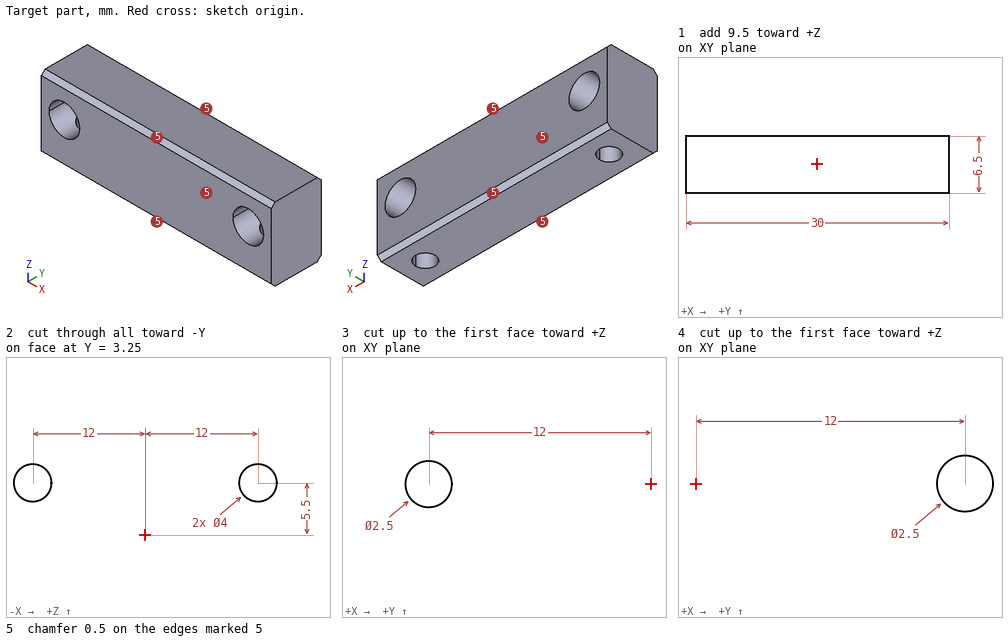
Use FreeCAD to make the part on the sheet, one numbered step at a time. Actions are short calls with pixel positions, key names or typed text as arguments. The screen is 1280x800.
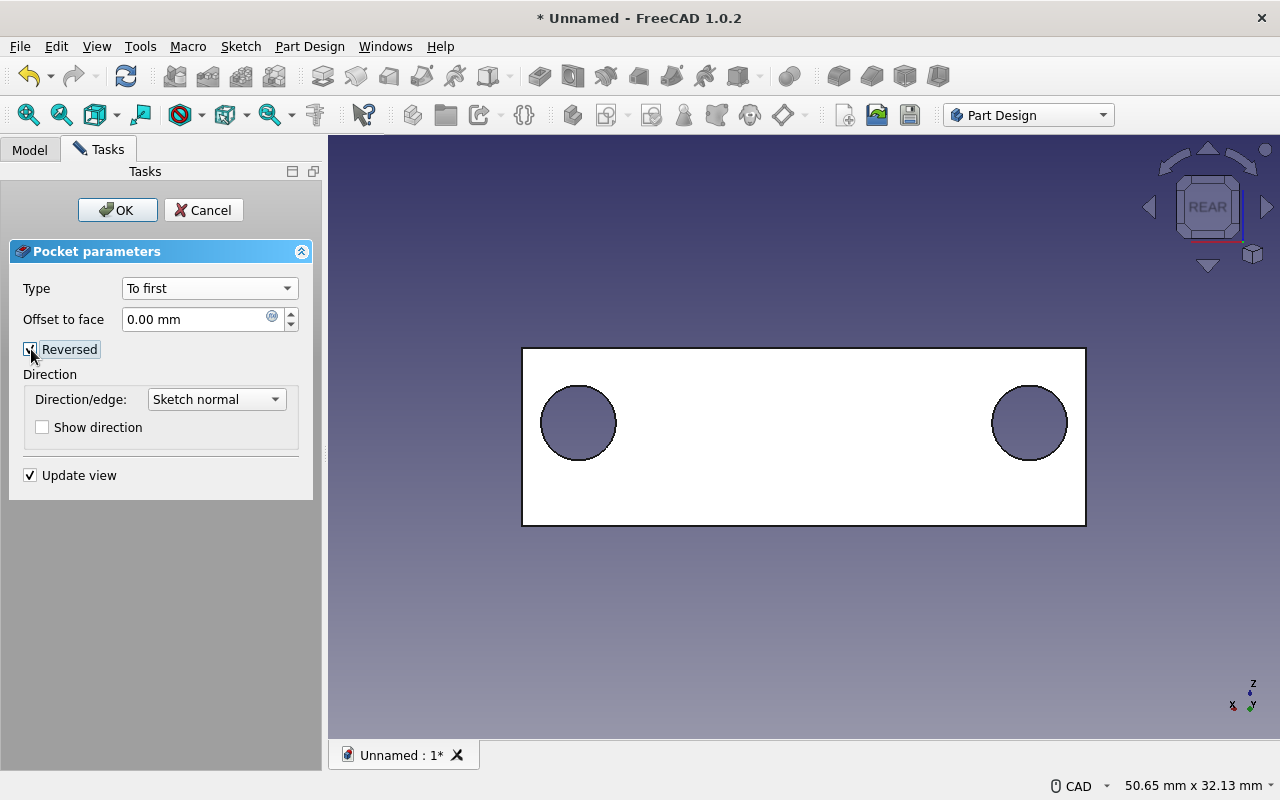
click(118, 210)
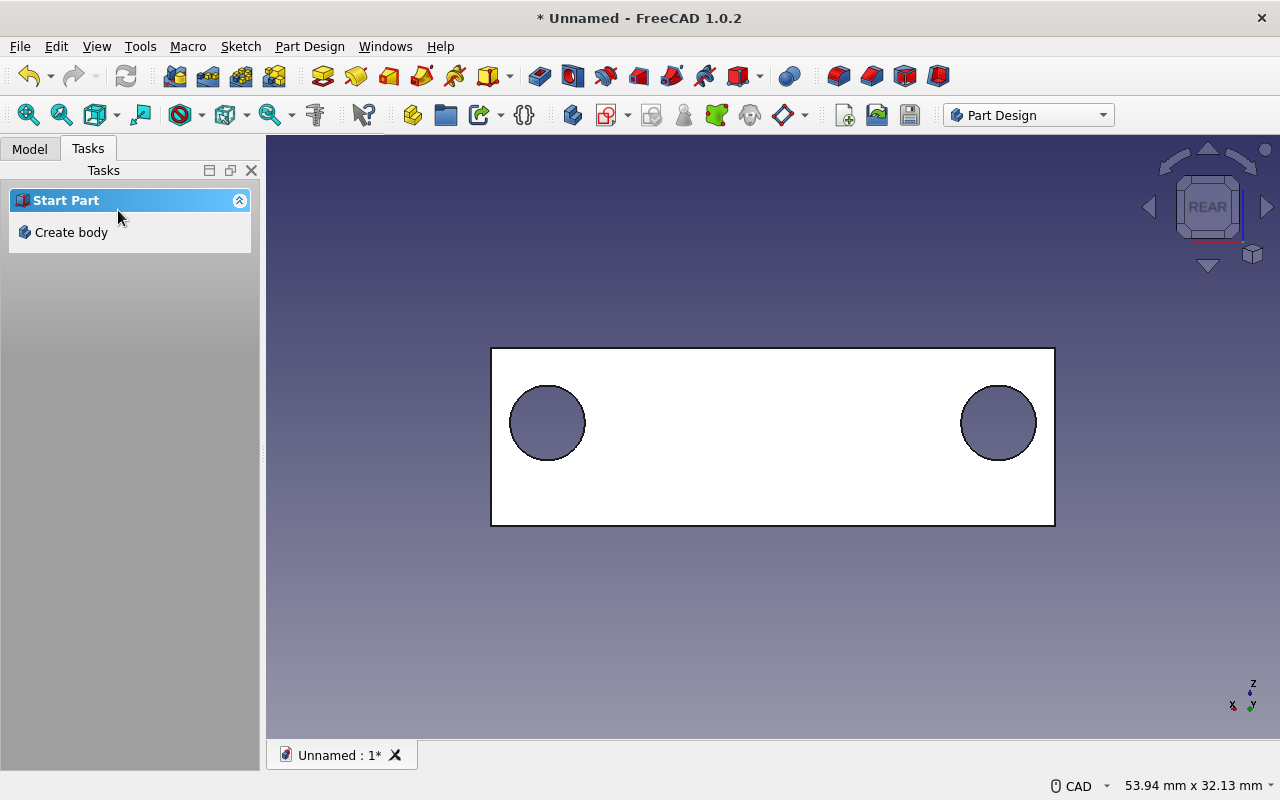
click(606, 116)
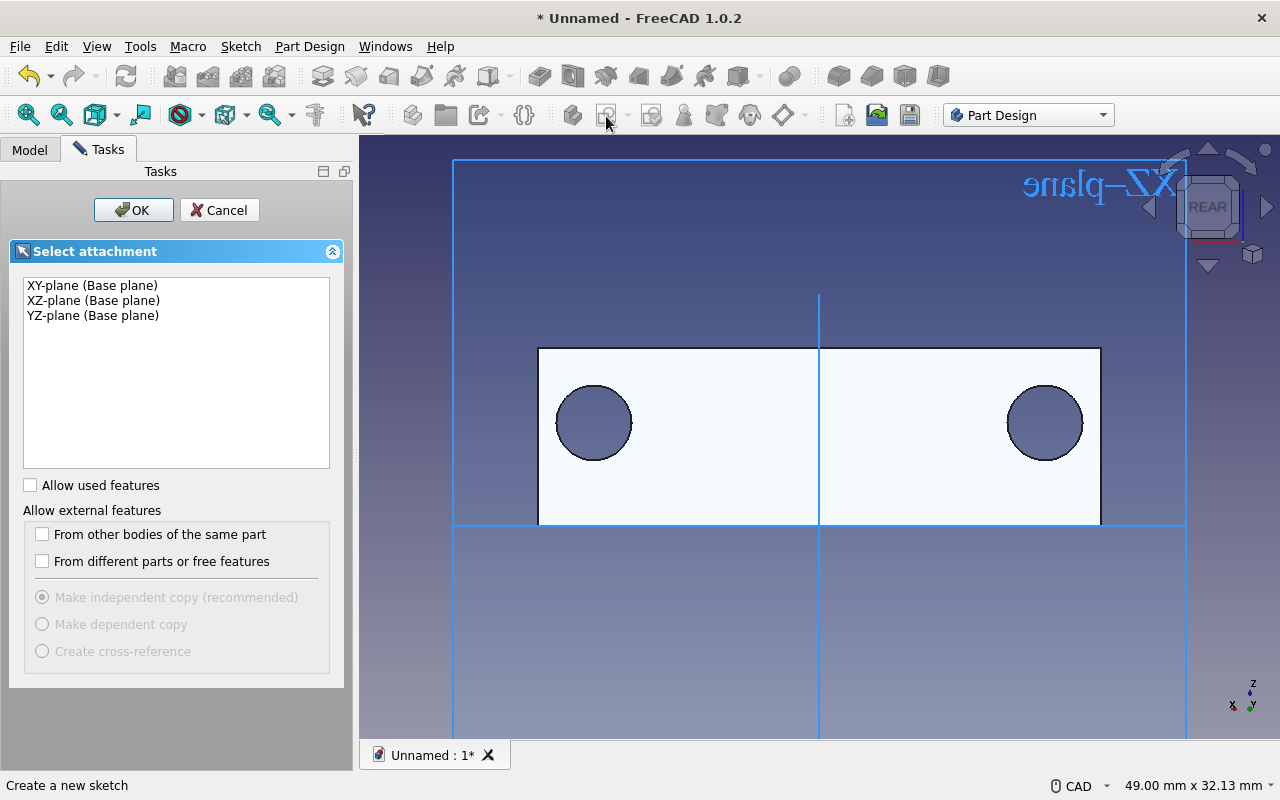
click(84, 286)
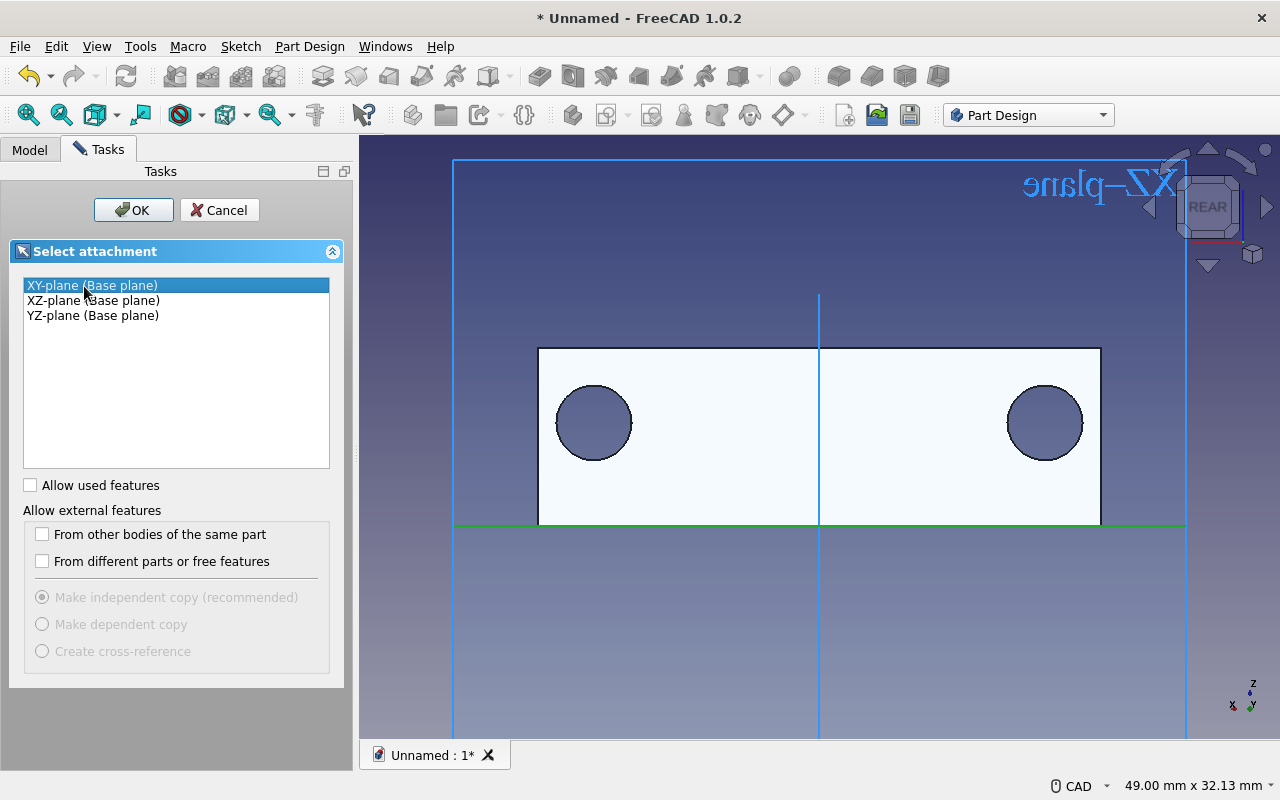
click(134, 210)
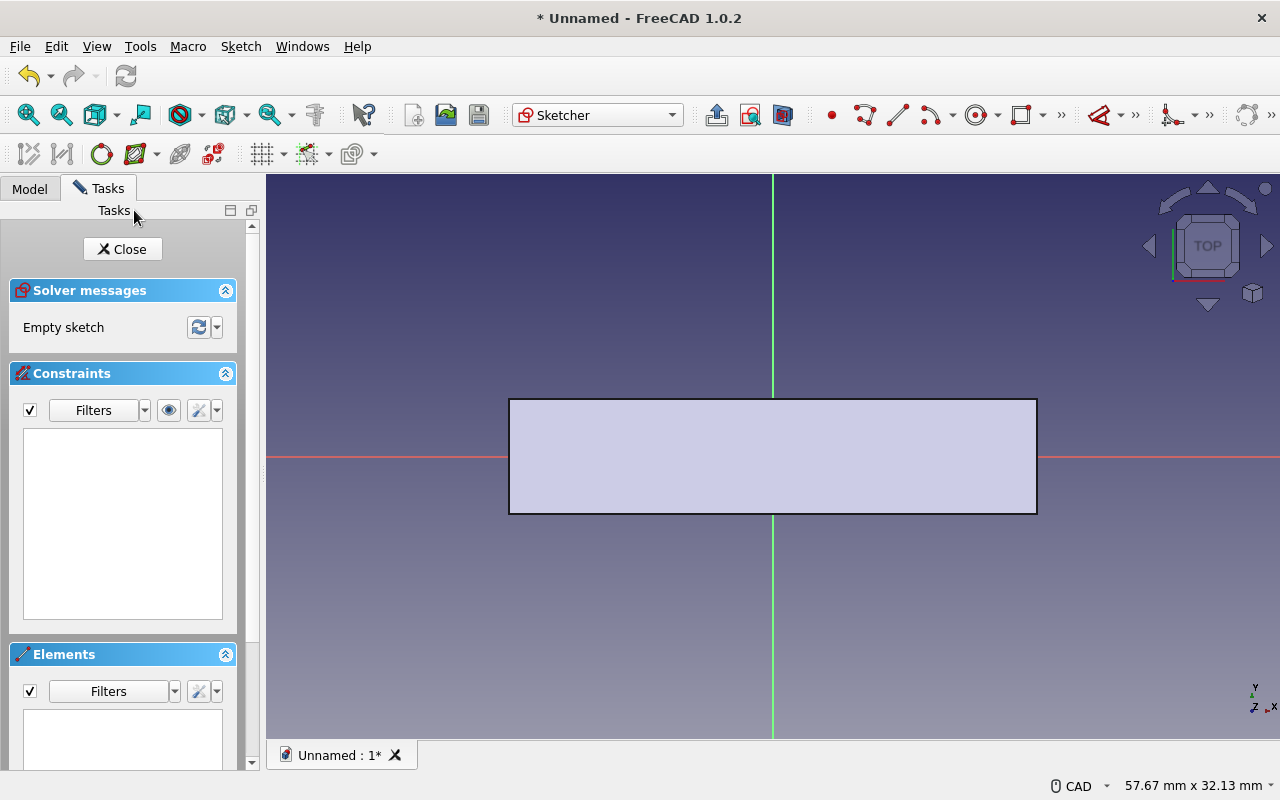
key(q)
key(s)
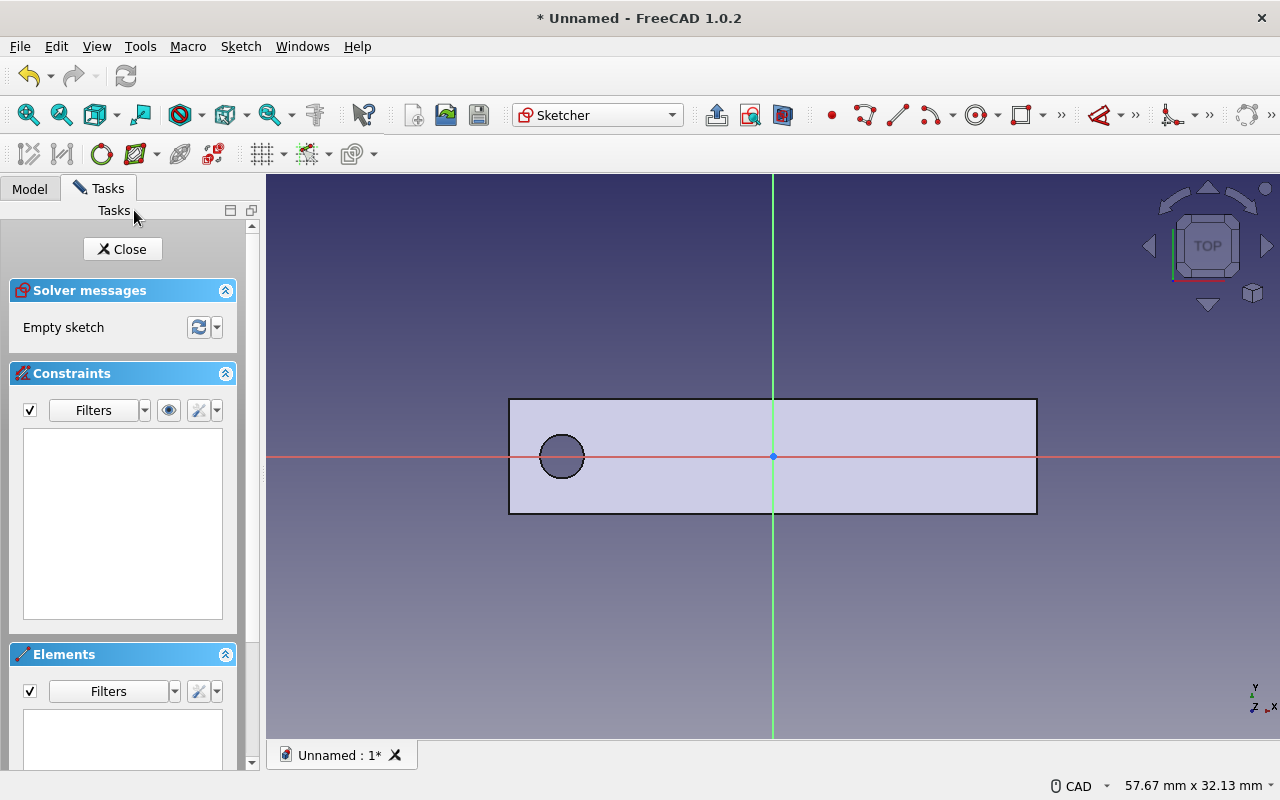
scroll(1019, 456, up, 11)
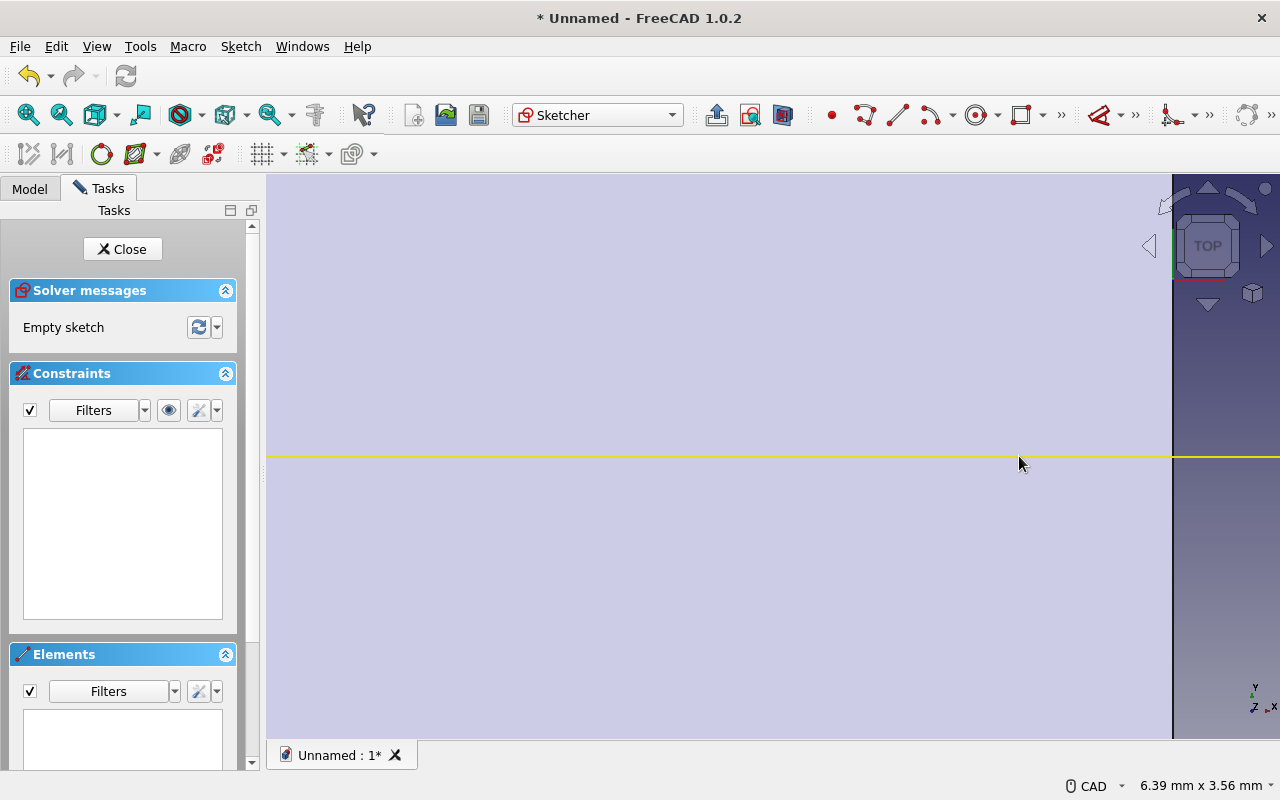
key(g)
key(c)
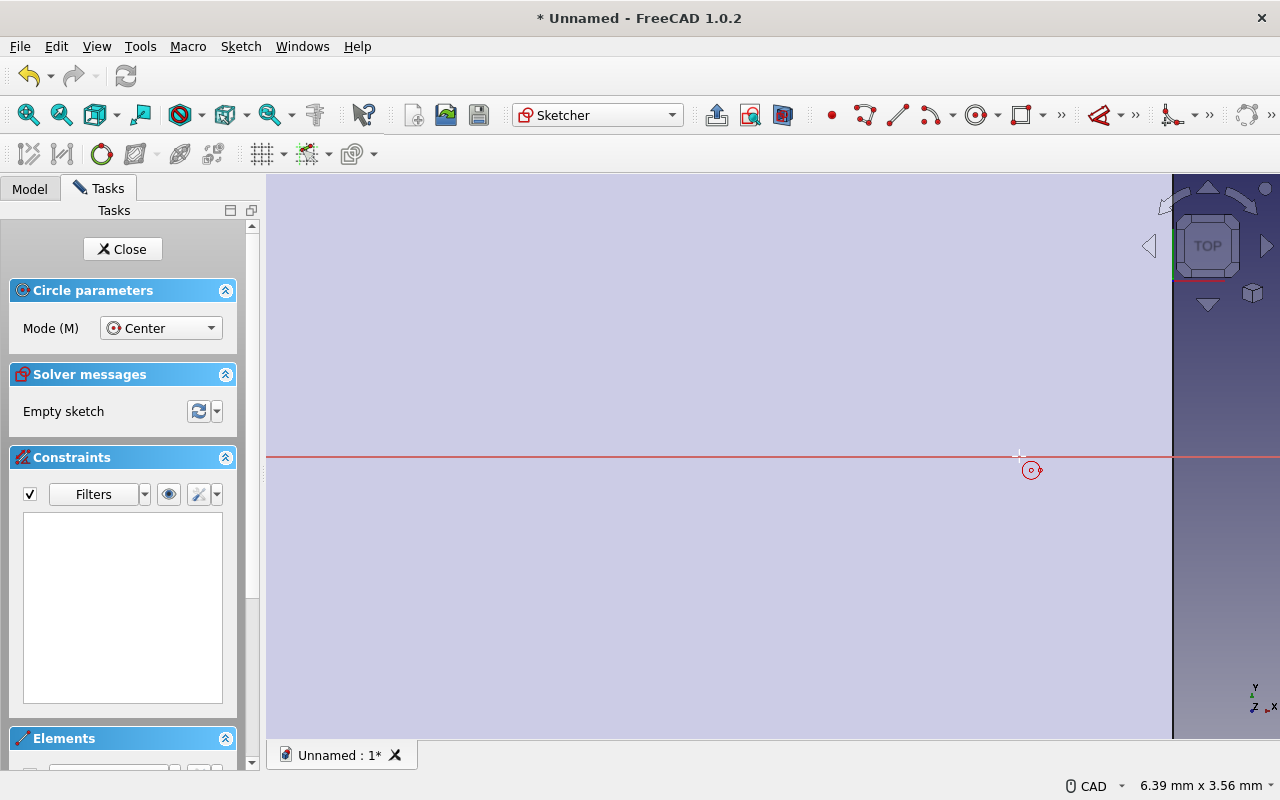
click(697, 456)
click(837, 316)
key(Escape)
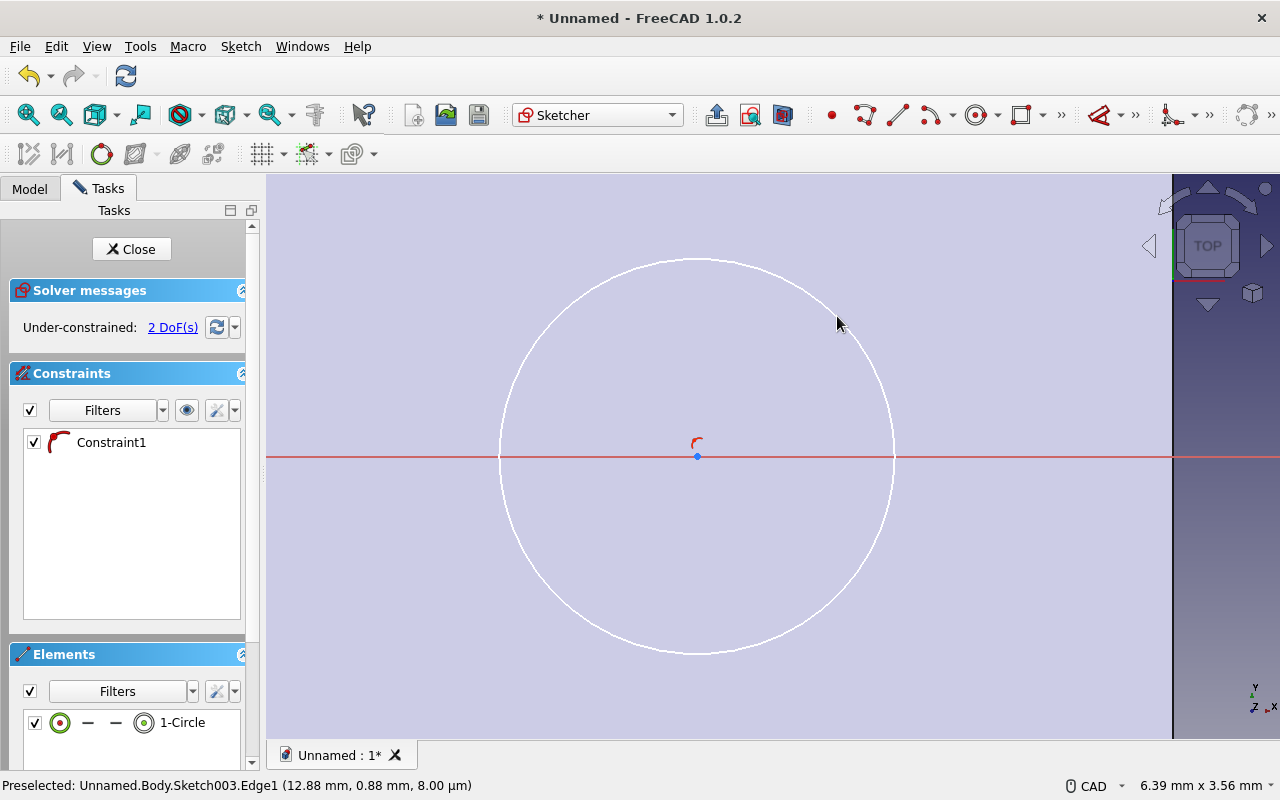
click(1098, 116)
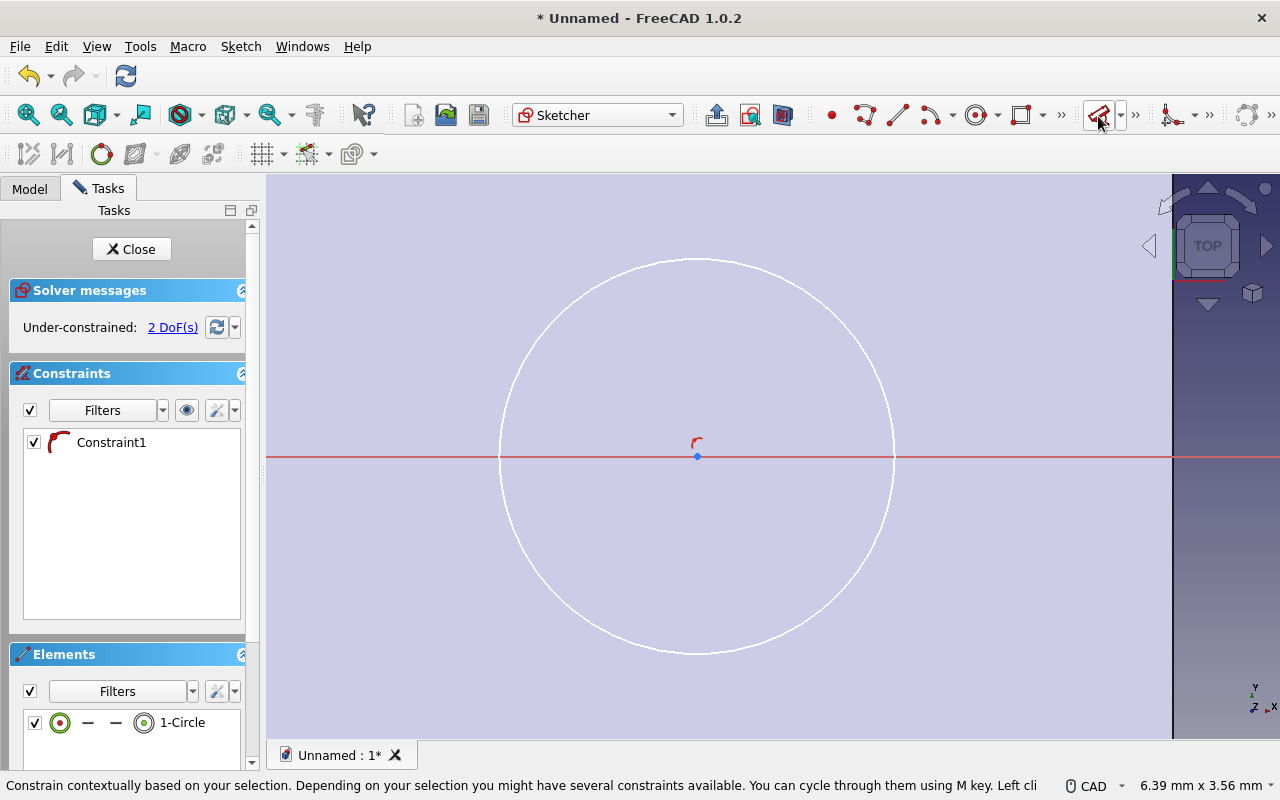
click(836, 316)
click(859, 293)